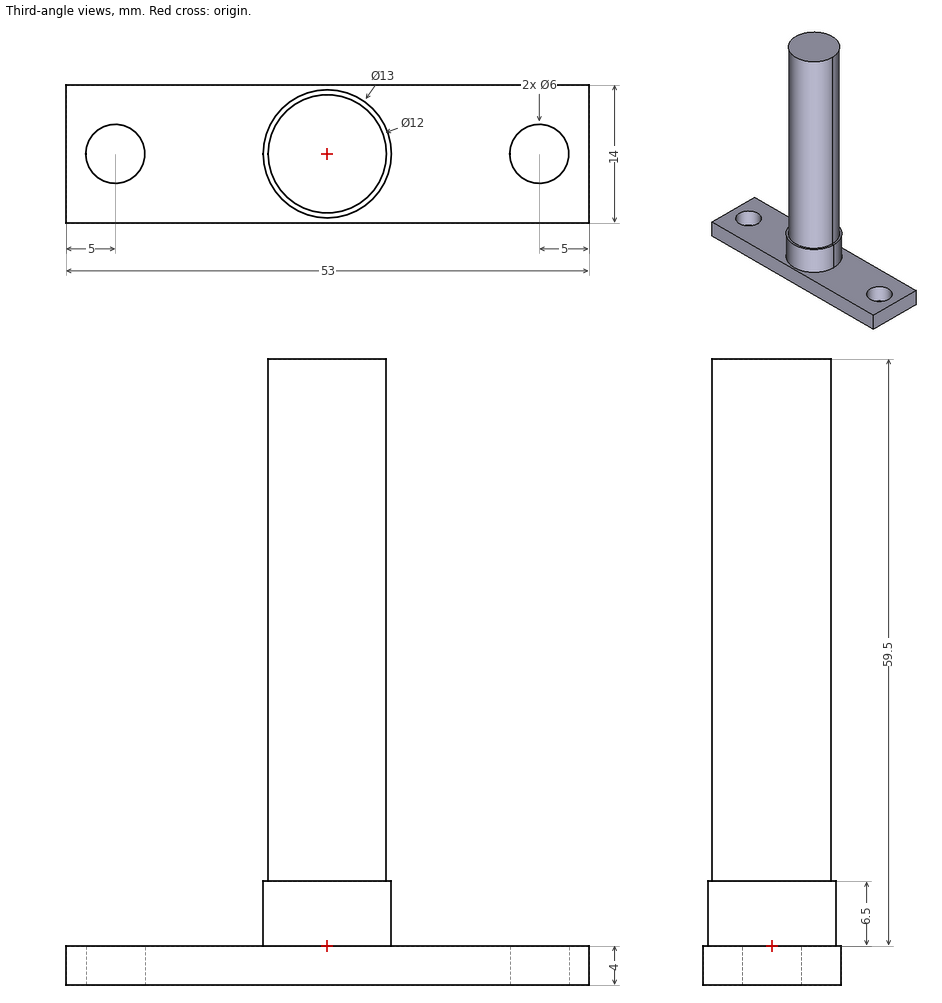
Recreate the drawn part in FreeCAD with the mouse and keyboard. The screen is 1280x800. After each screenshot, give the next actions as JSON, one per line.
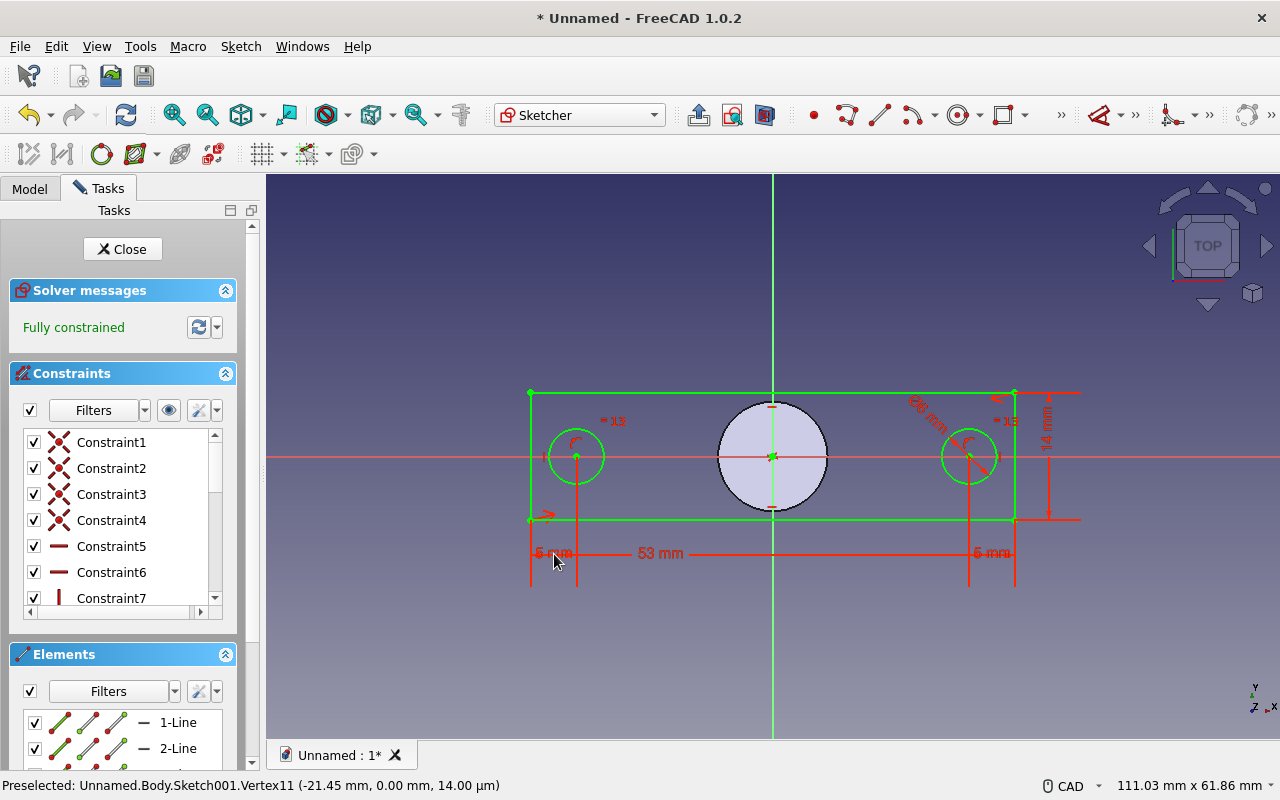
{"action": "left_click", "coordinate": [123, 249]}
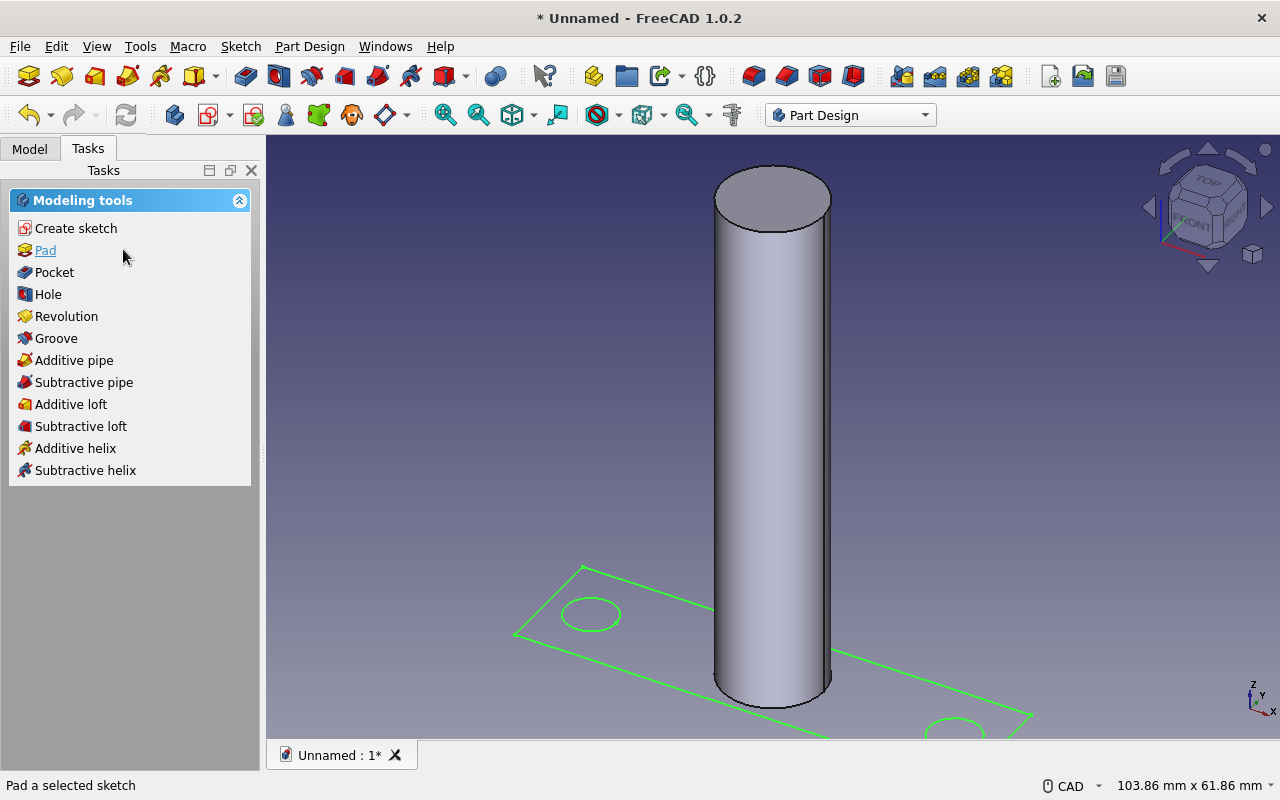
{"action": "left_click", "coordinate": [29, 76]}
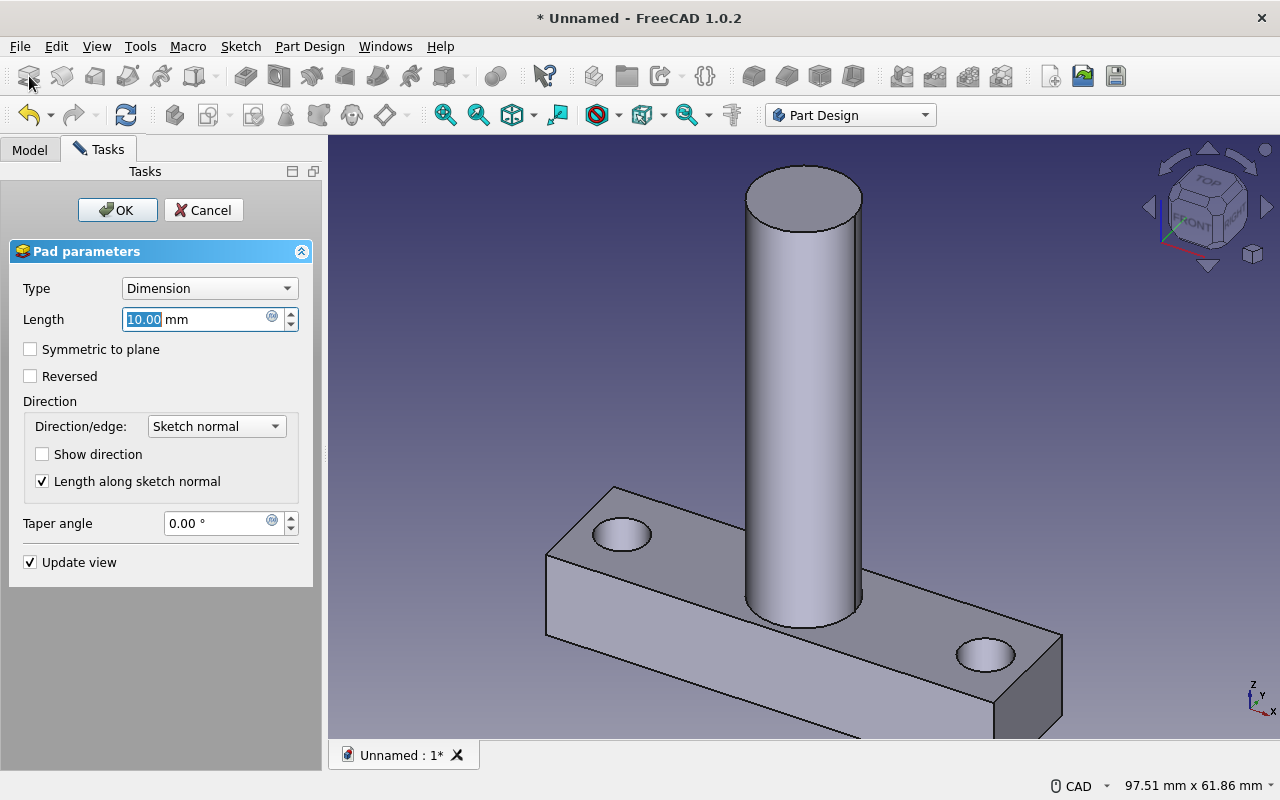
{"action": "type", "text": "4"}
{"action": "key", "text": "Tab"}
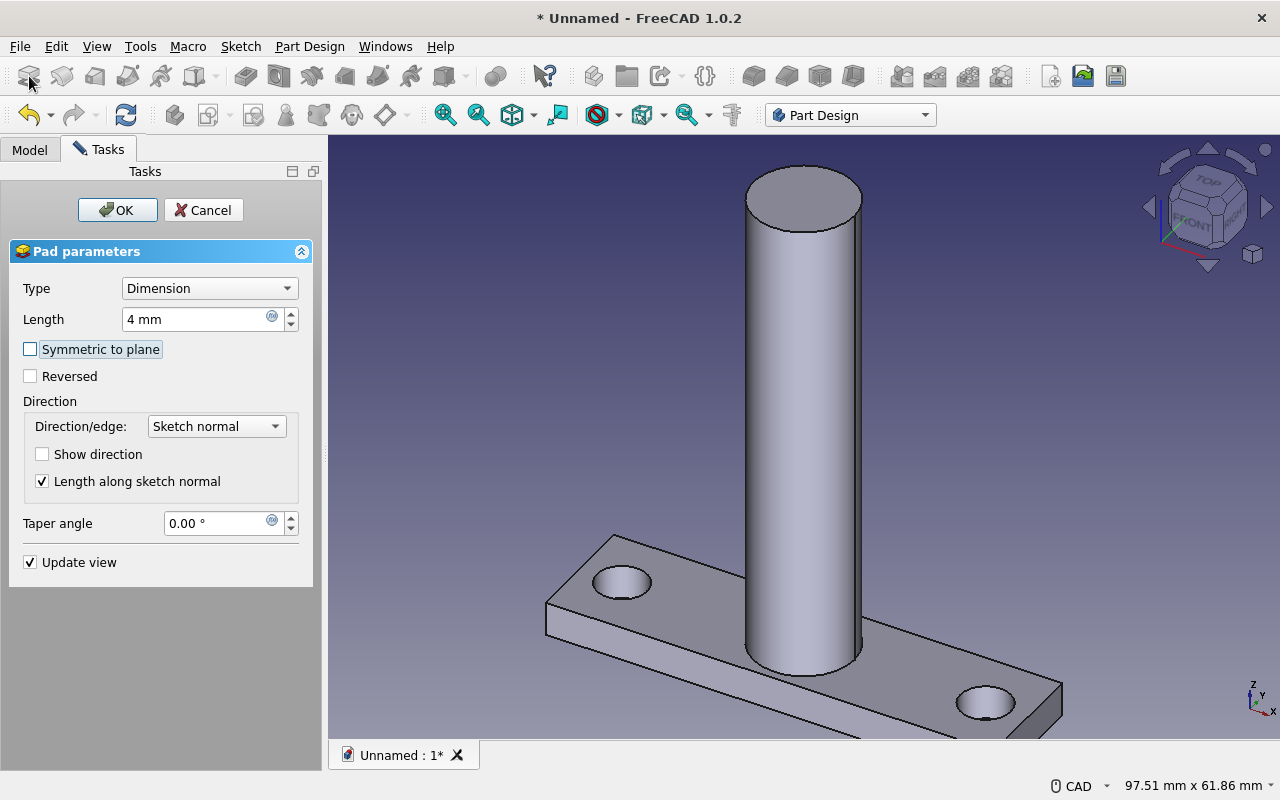
{"action": "left_click", "coordinate": [31, 376]}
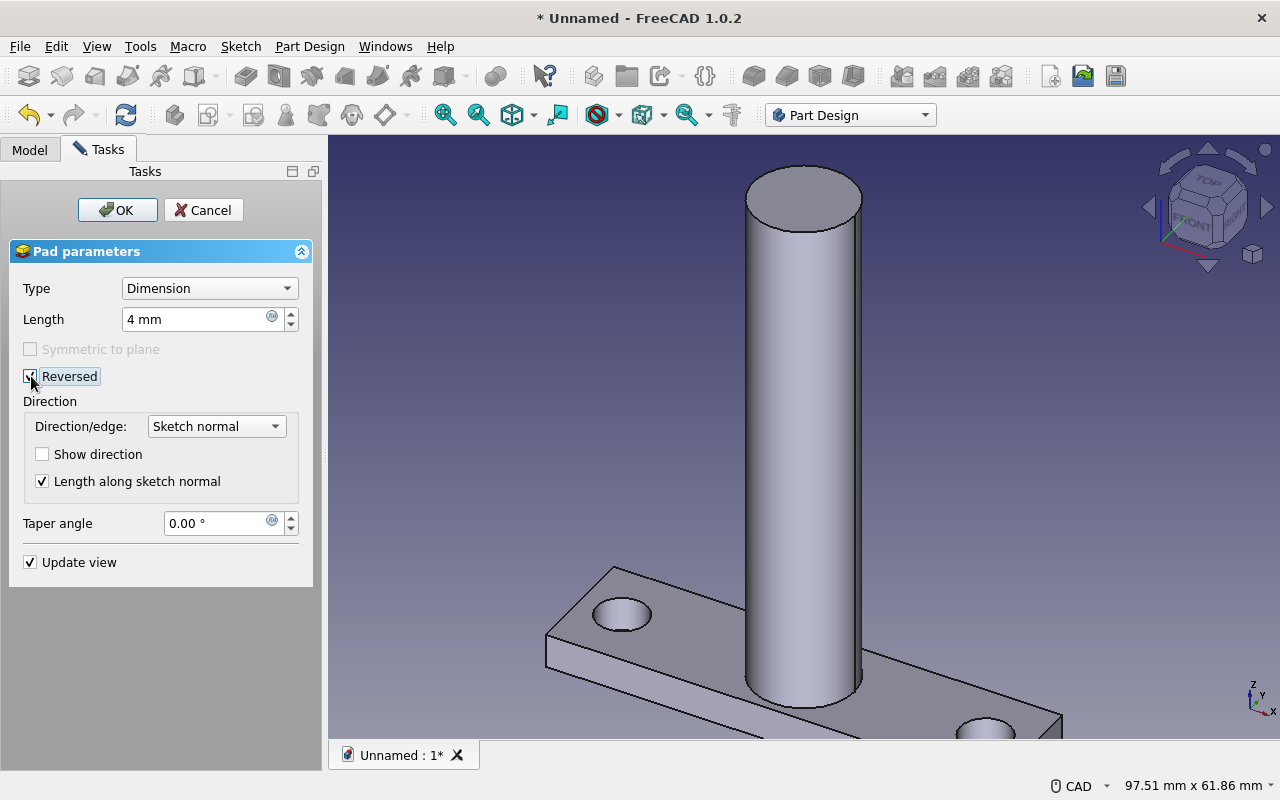
{"action": "left_click", "coordinate": [118, 210]}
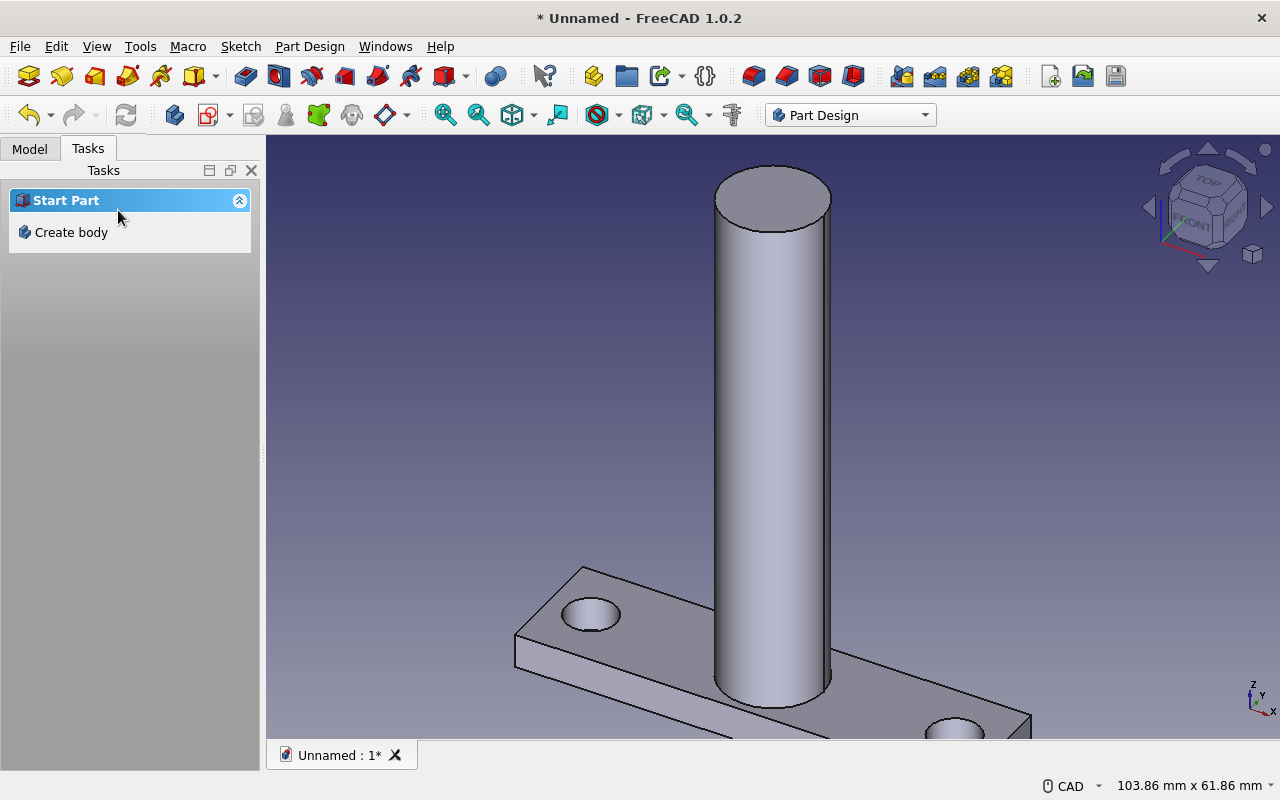
{"action": "key", "text": "v f"}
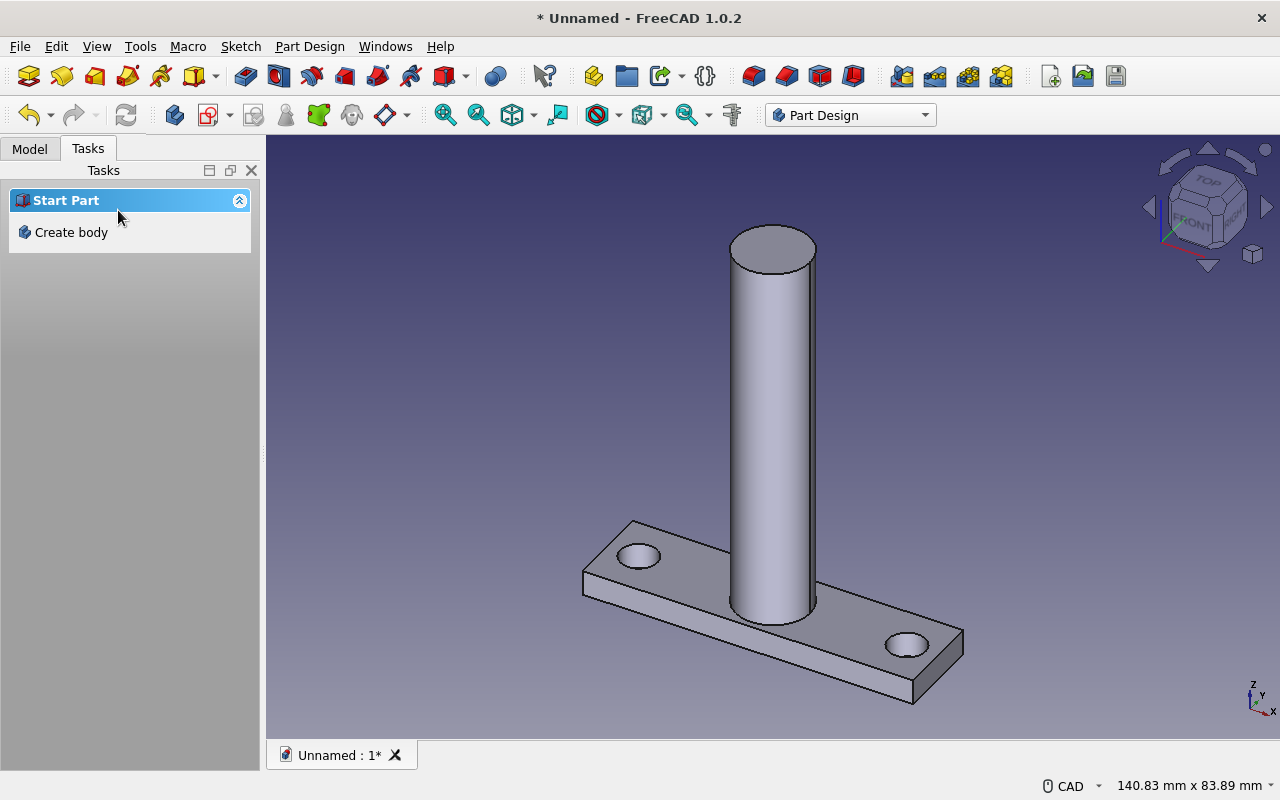
{"action": "left_click", "coordinate": [208, 116]}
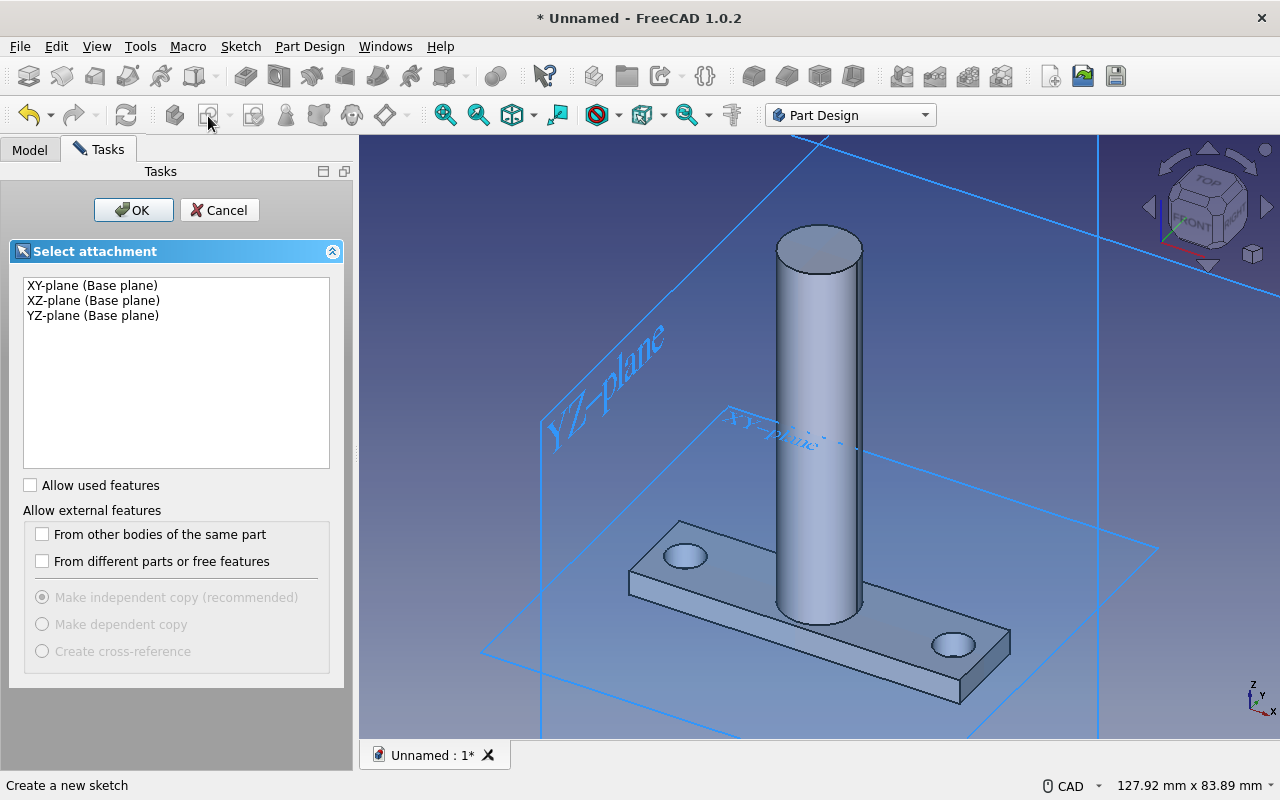
{"action": "left_click", "coordinate": [84, 286]}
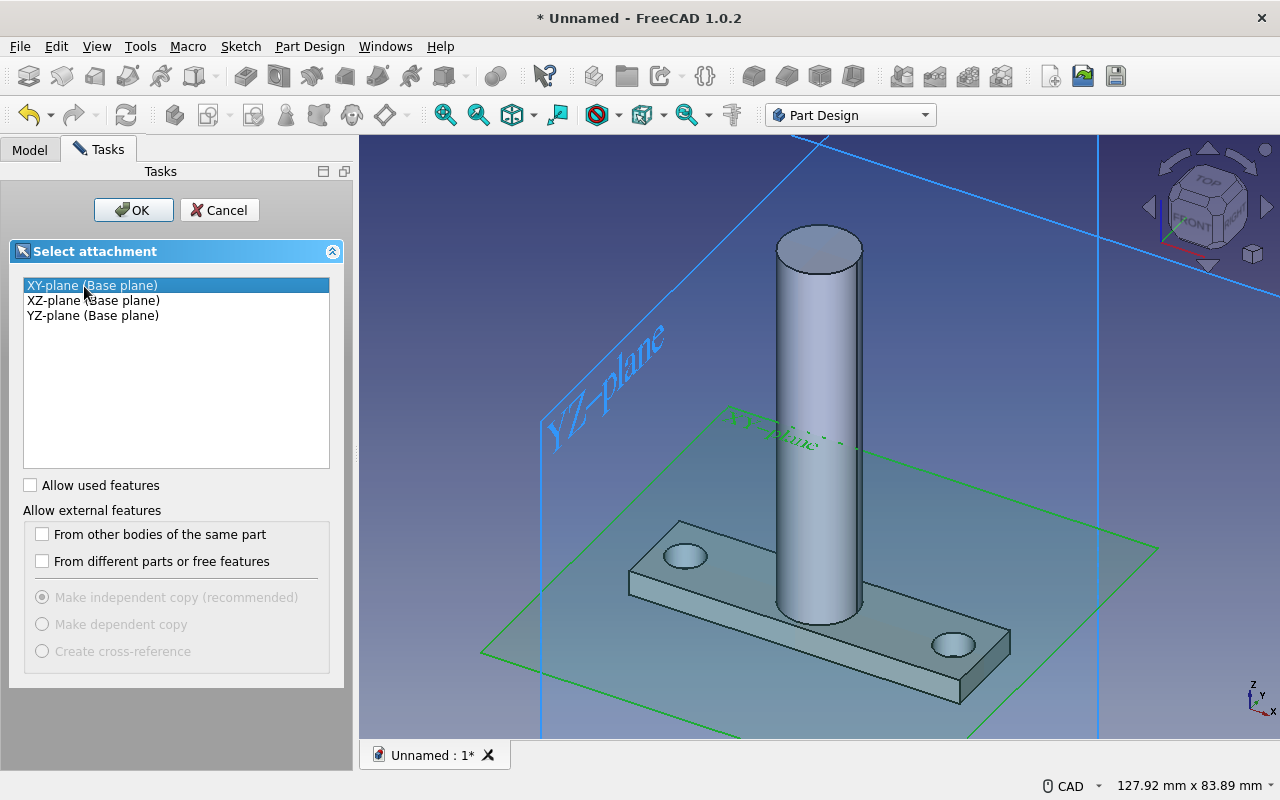
{"action": "left_click", "coordinate": [134, 210]}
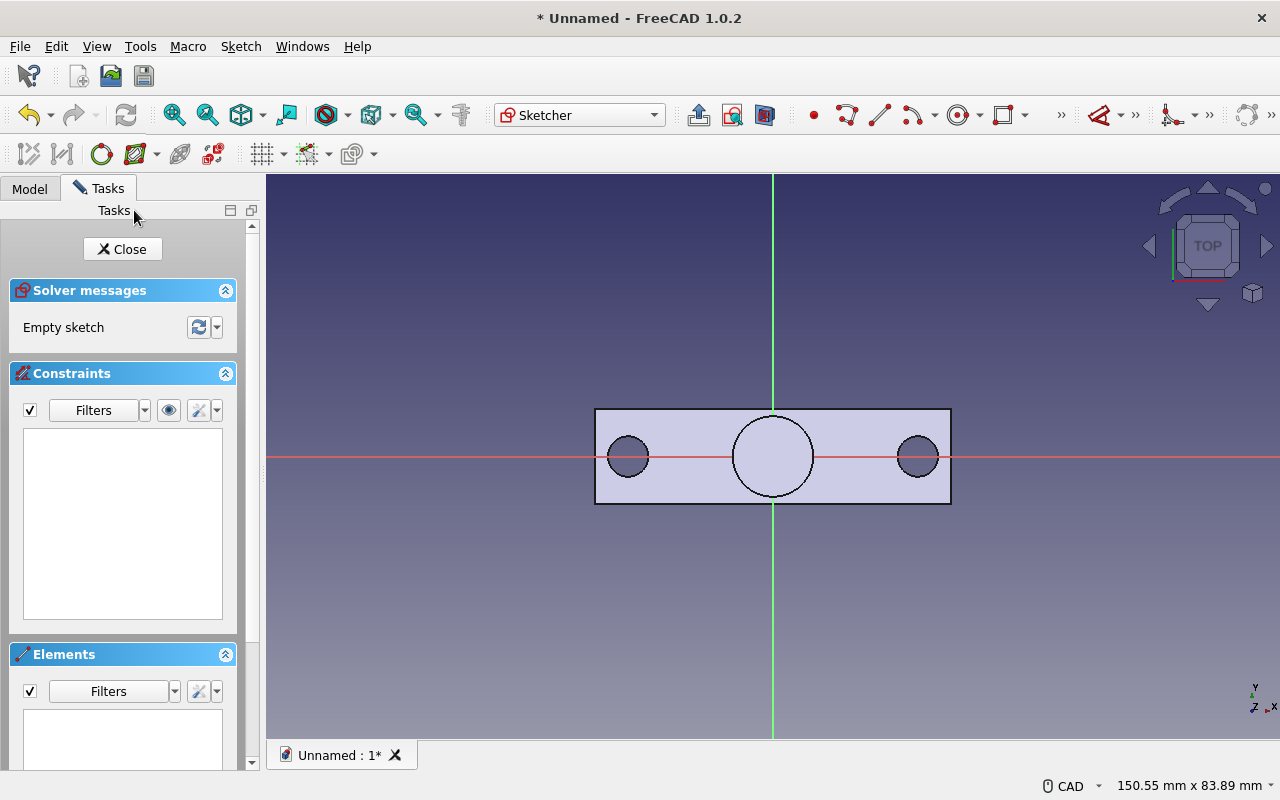
{"action": "left_click", "coordinate": [765, 116]}